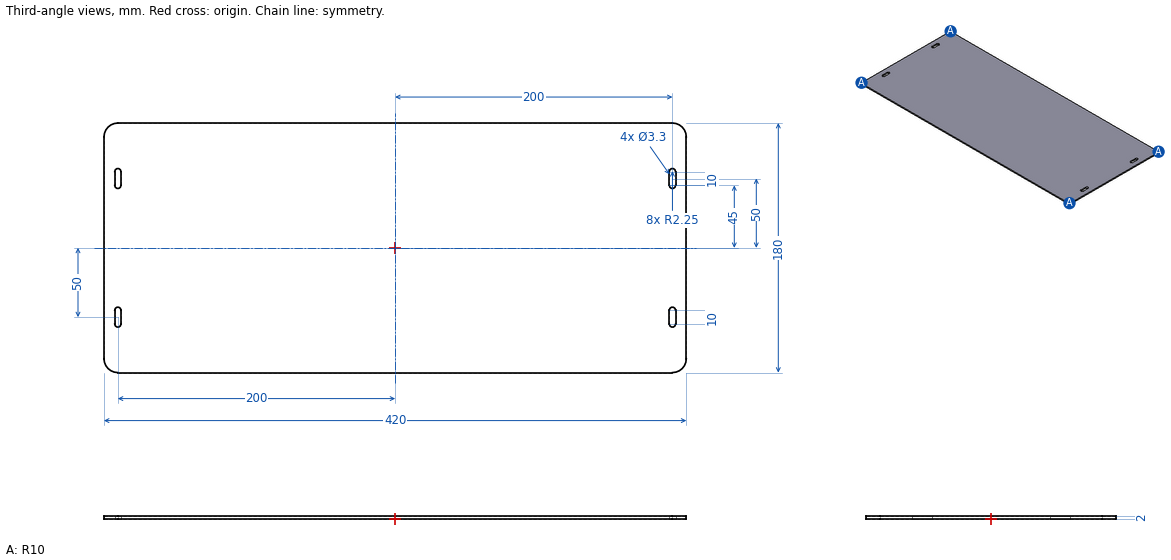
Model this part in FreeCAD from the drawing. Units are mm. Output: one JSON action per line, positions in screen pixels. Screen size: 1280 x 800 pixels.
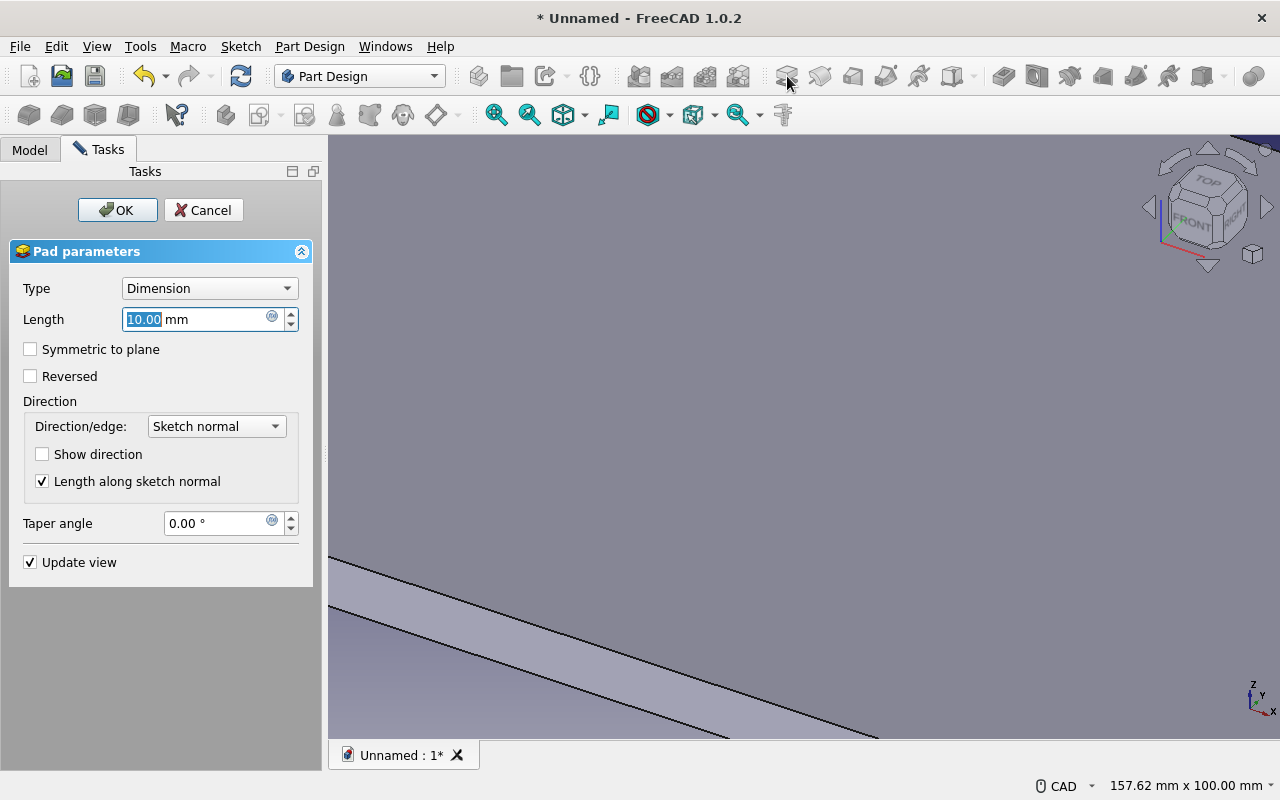
{"action": "type", "text": "2"}
{"action": "key", "text": "Tab"}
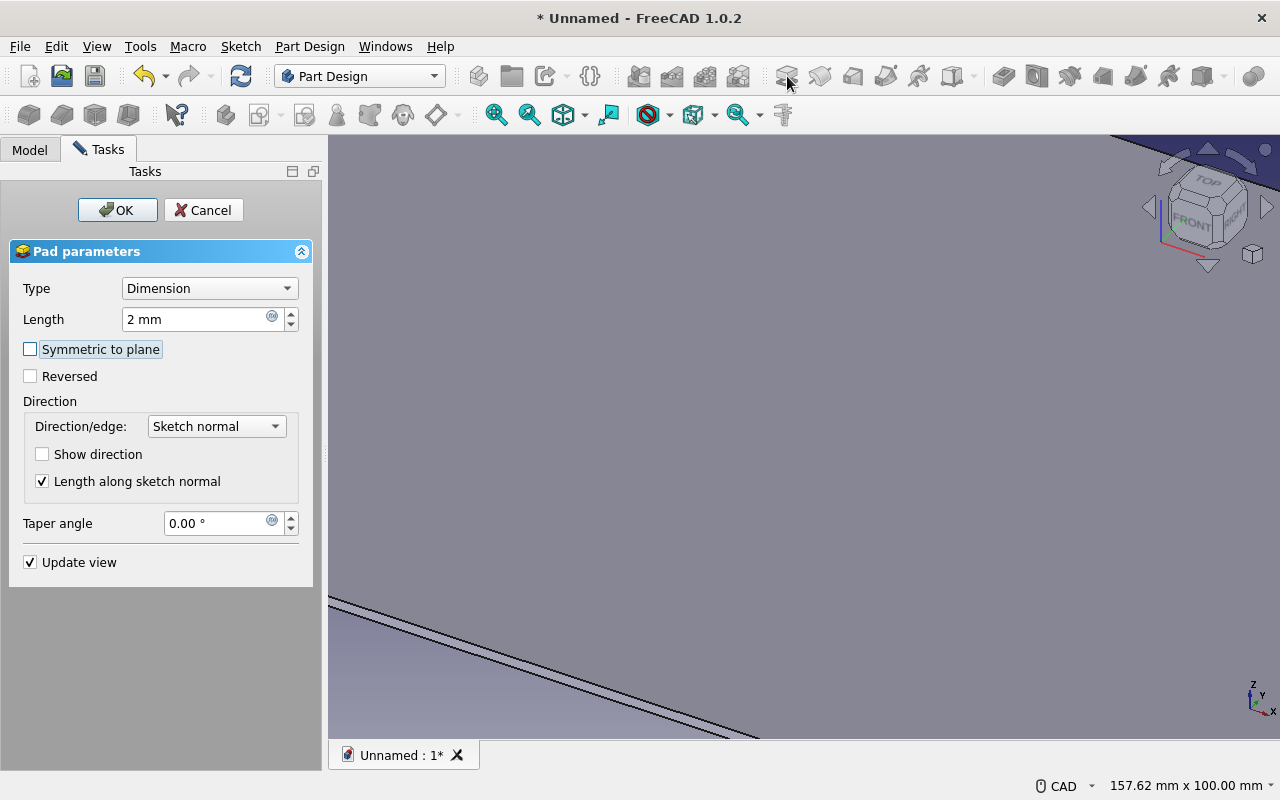
{"action": "left_click", "coordinate": [118, 210]}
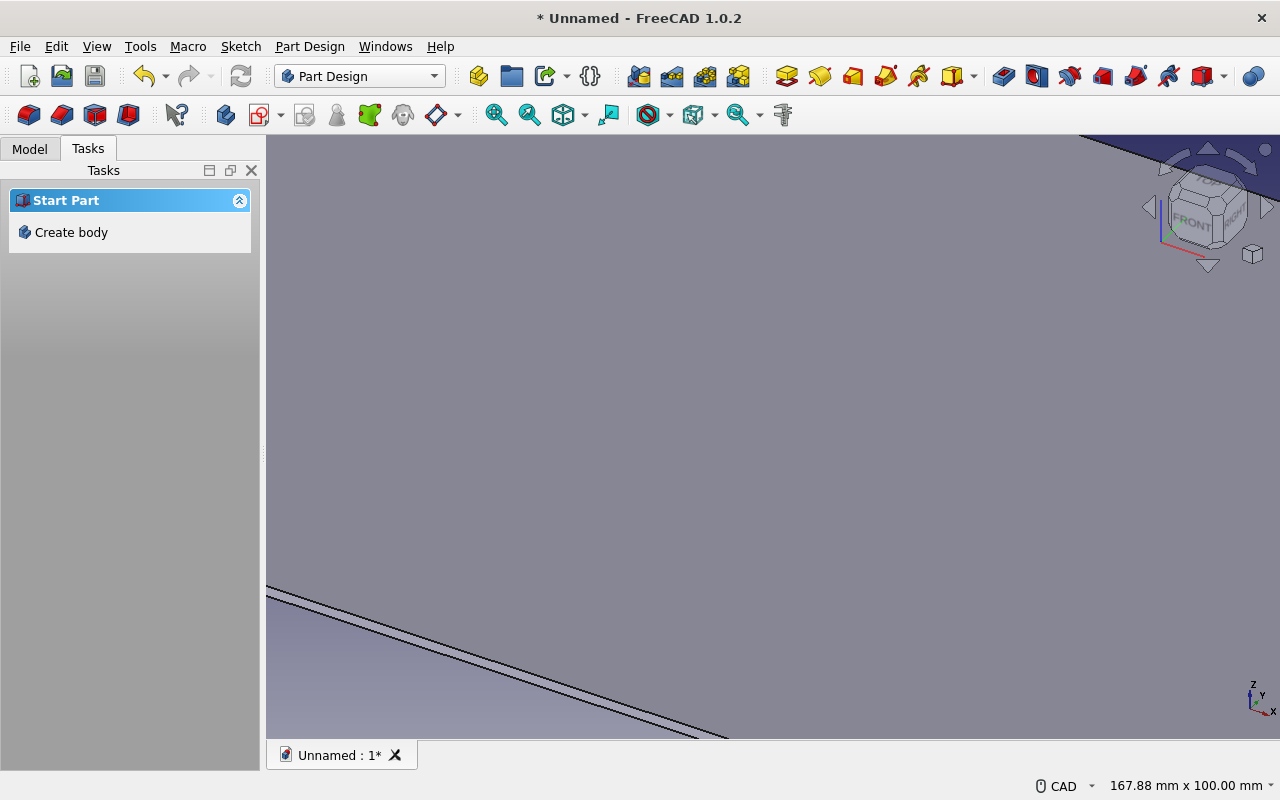
{"action": "key", "text": "v f"}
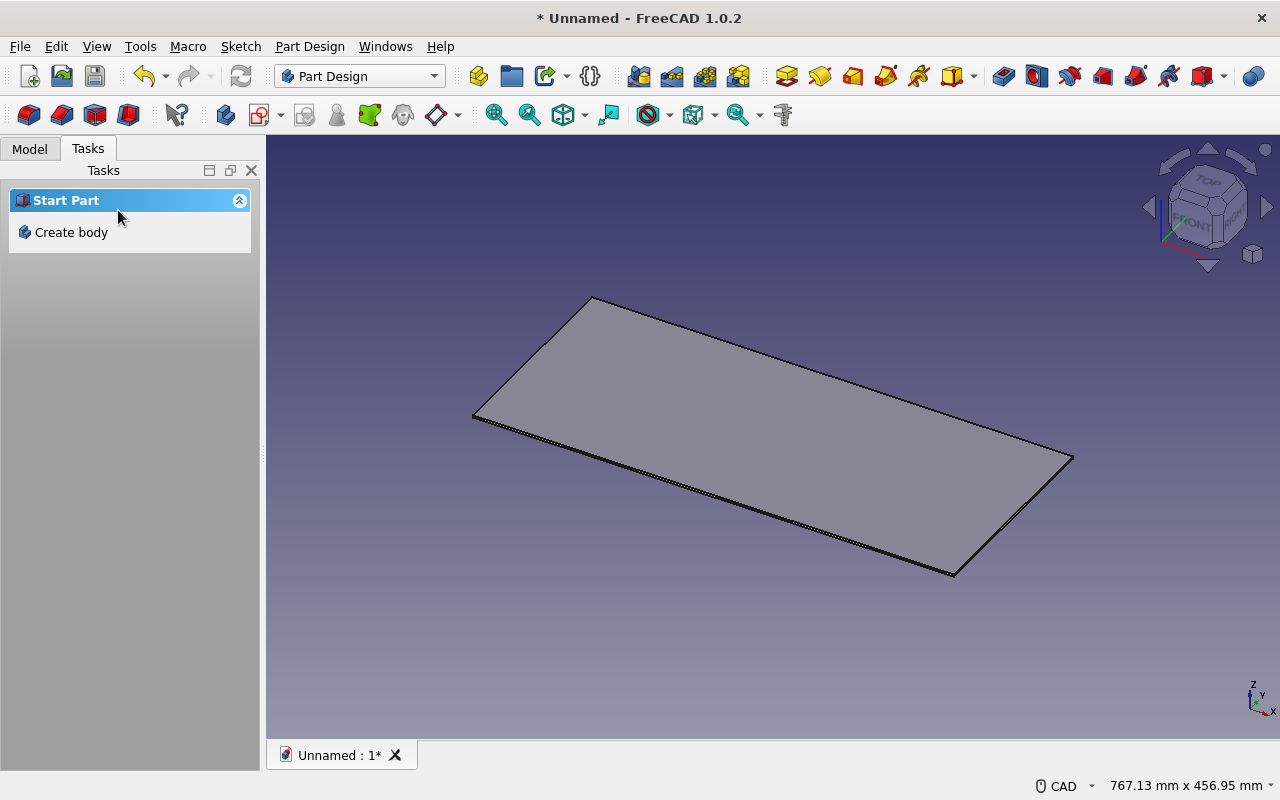
{"action": "left_click", "coordinate": [910, 480]}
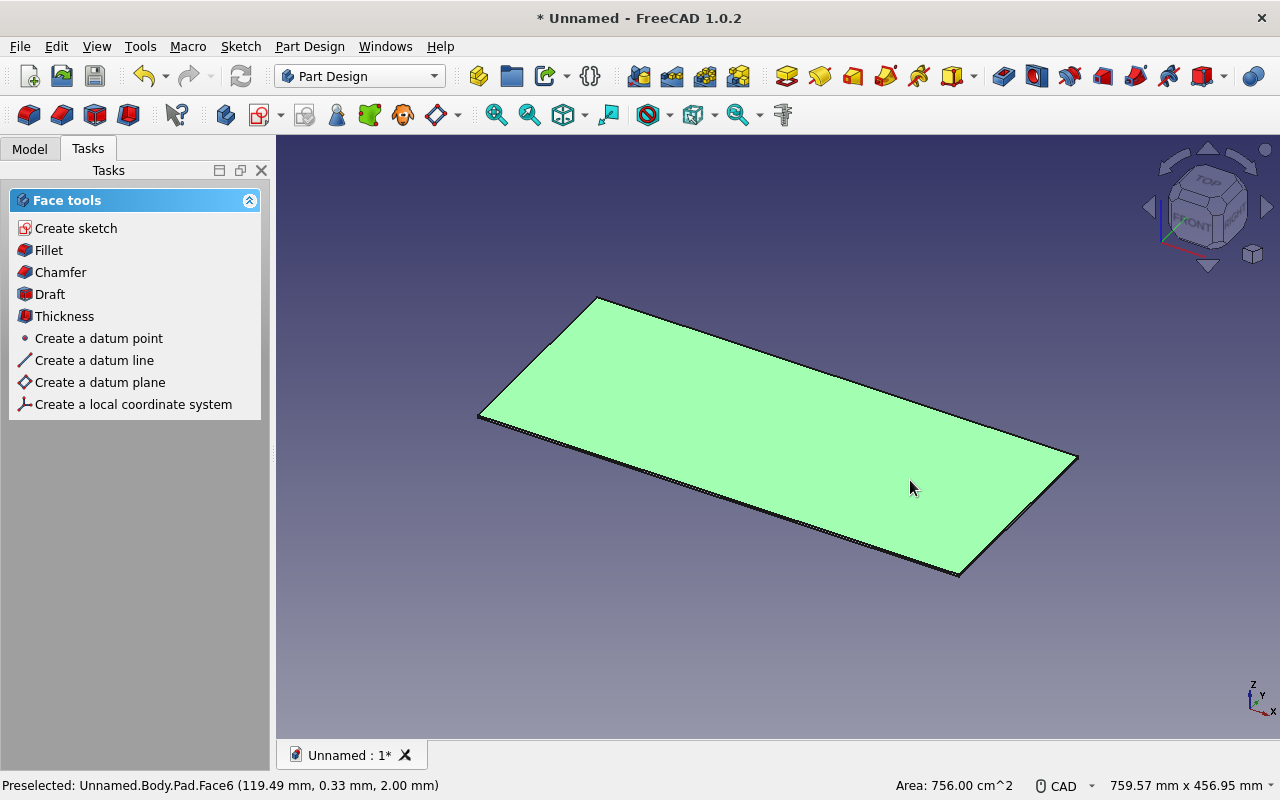
{"action": "left_click", "coordinate": [258, 116]}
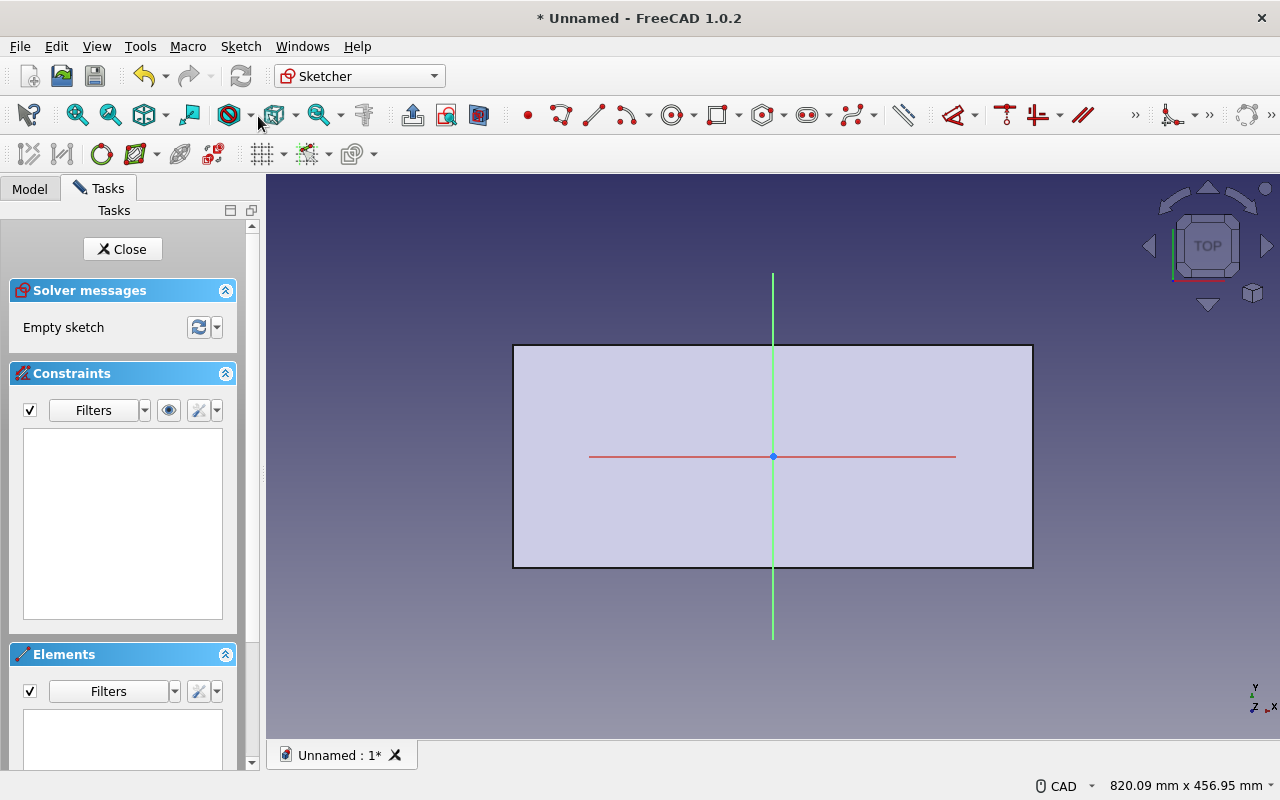
{"action": "left_click", "coordinate": [672, 116]}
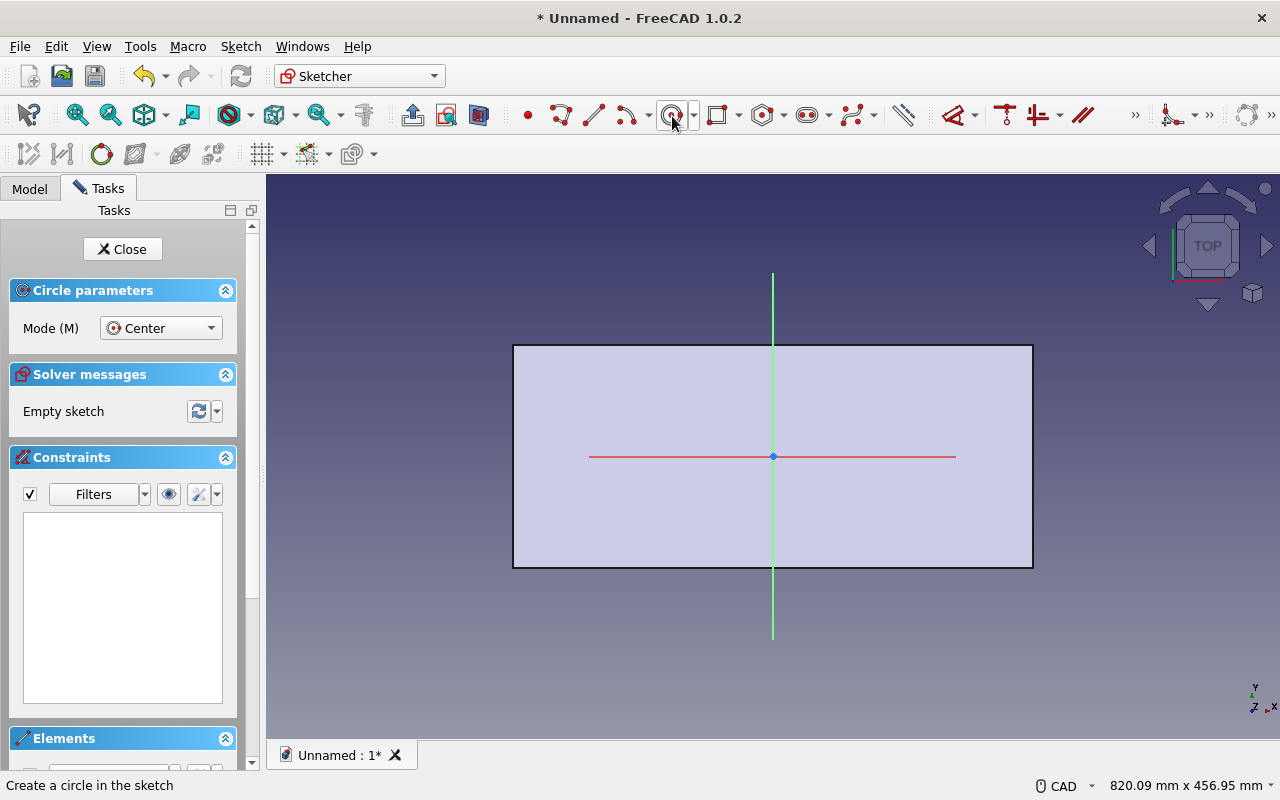
{"action": "scroll", "coordinate": [1020, 395], "scroll_direction": "up", "scroll_amount": 13}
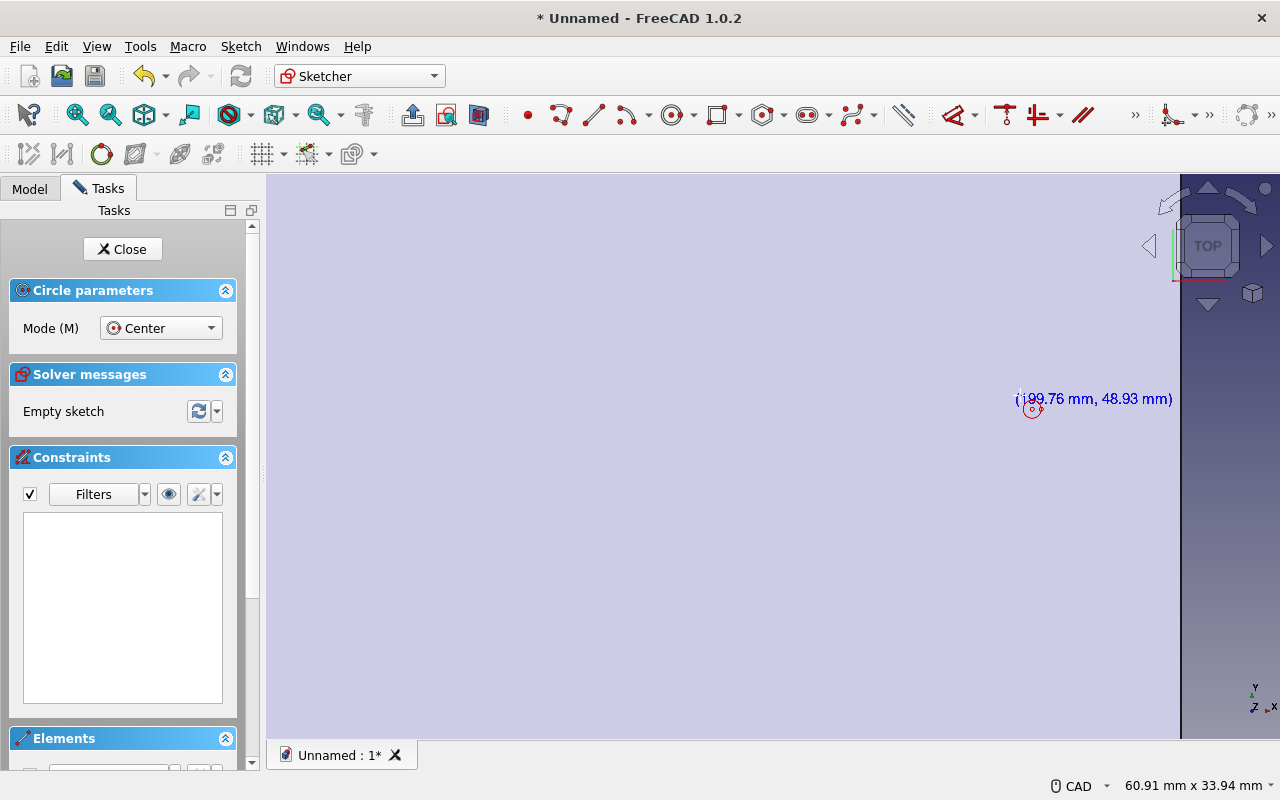
{"action": "scroll", "coordinate": [1006, 381], "scroll_direction": "down", "scroll_amount": 12}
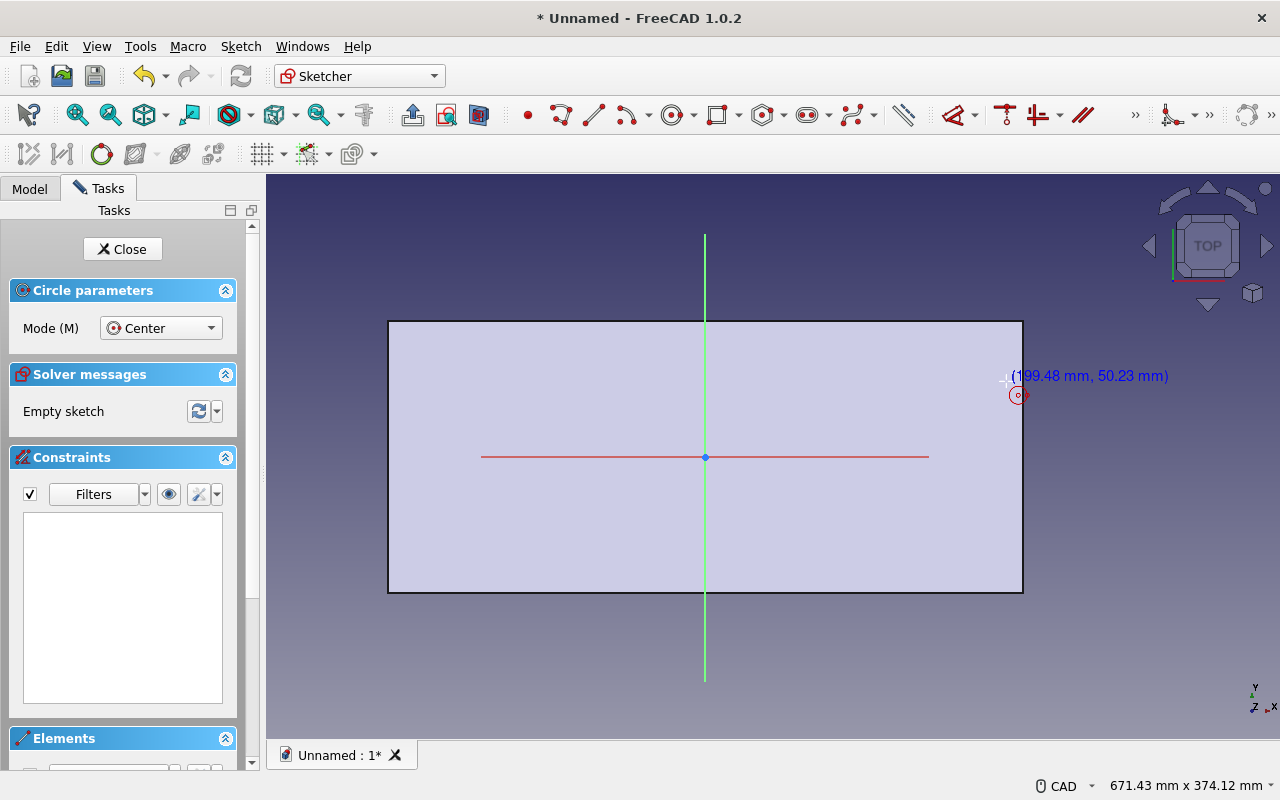
{"action": "left_click", "coordinate": [1007, 382]}
{"action": "mouse_move", "coordinate": [1009, 380]}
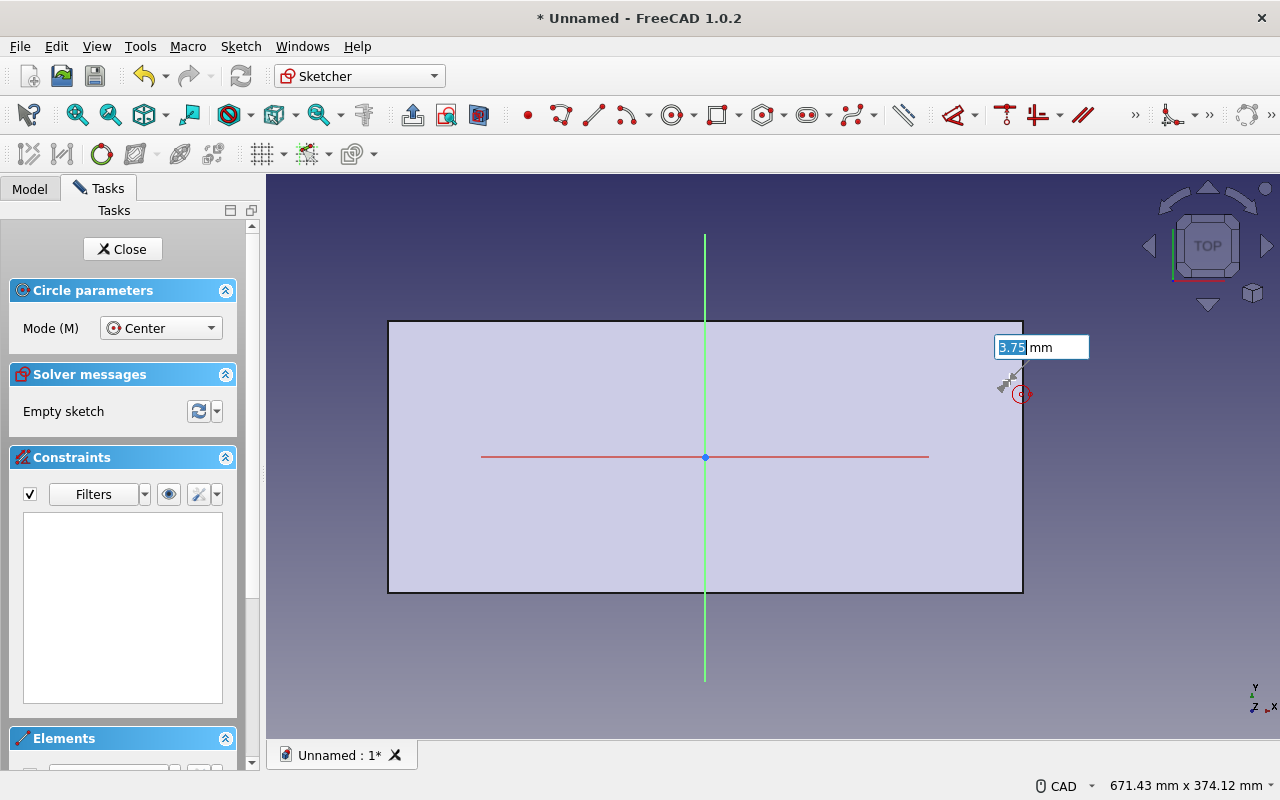
{"action": "type", "text": "3.3"}
{"action": "key", "text": "Return"}